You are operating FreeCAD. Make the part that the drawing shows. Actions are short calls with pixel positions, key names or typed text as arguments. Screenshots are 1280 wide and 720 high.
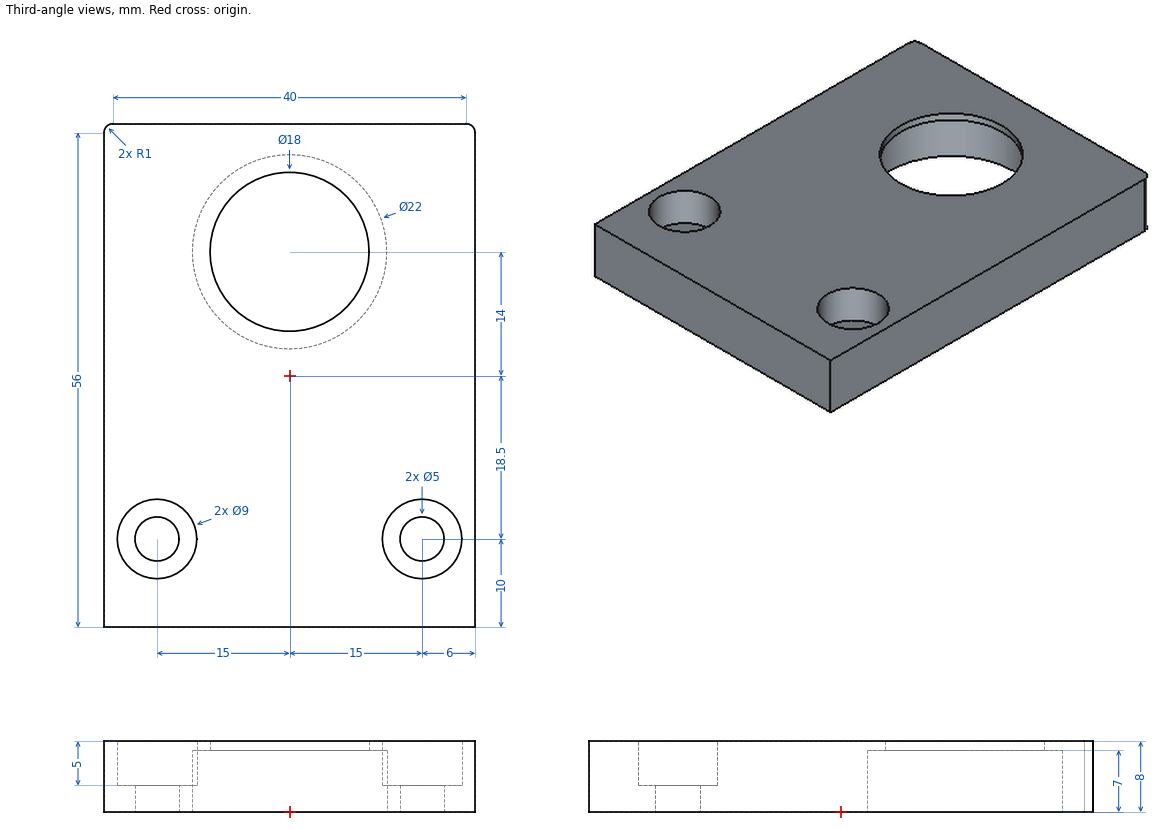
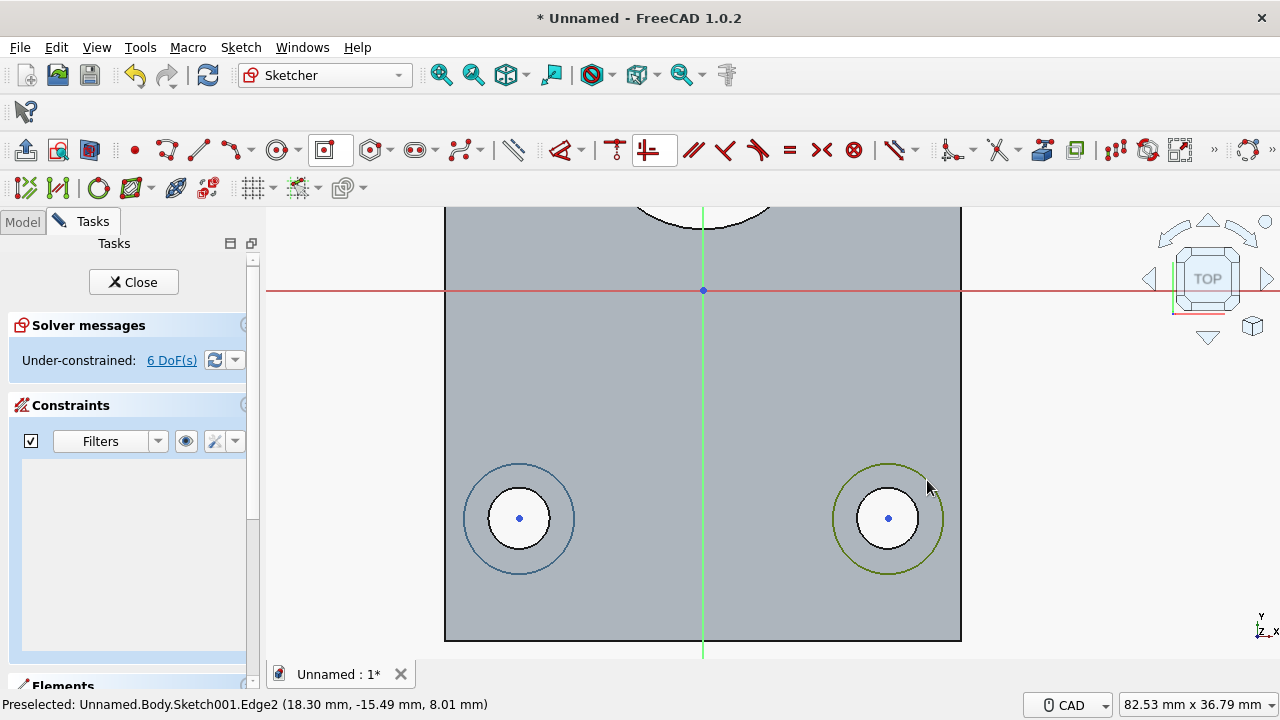
click(790, 150)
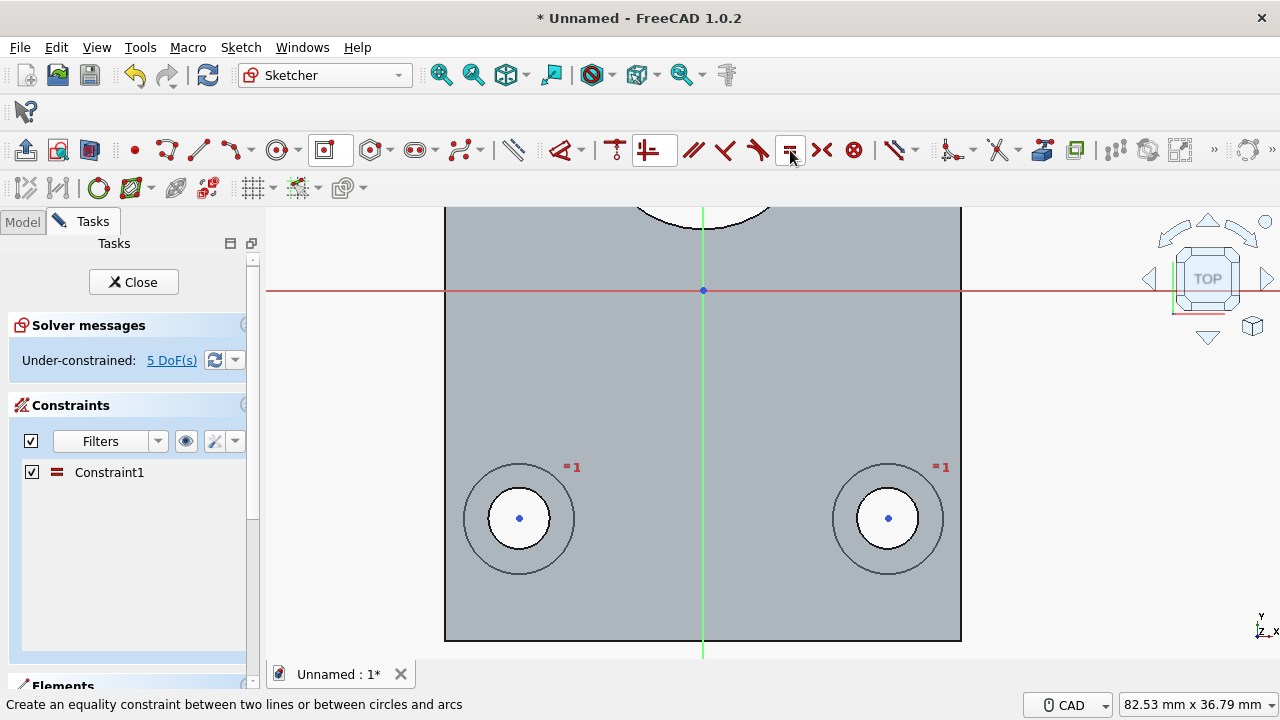
click(519, 519)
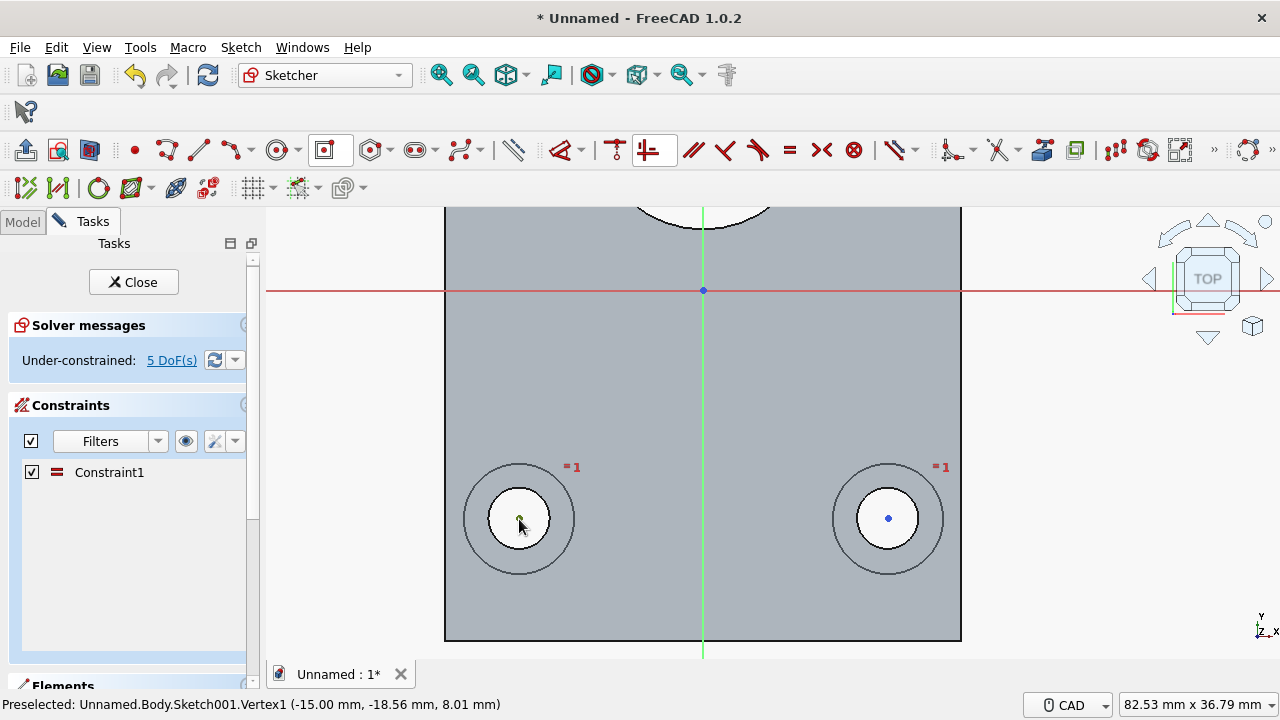
click(888, 519)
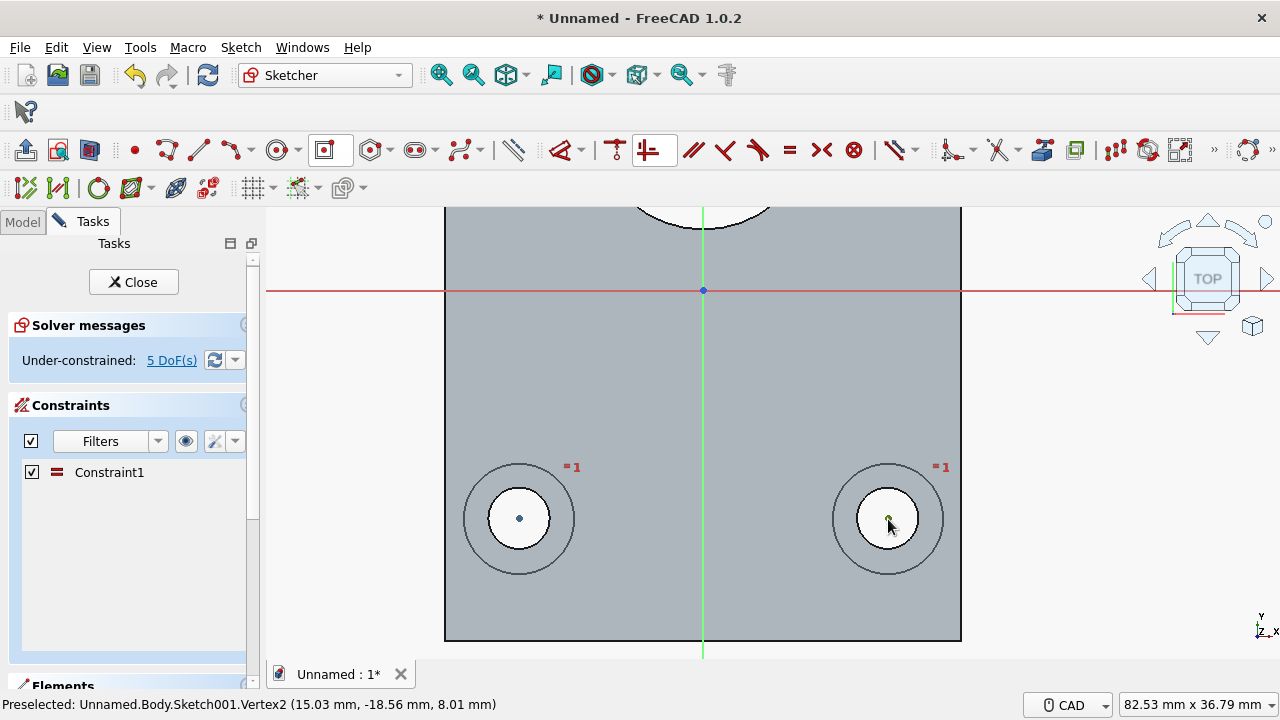
click(672, 150)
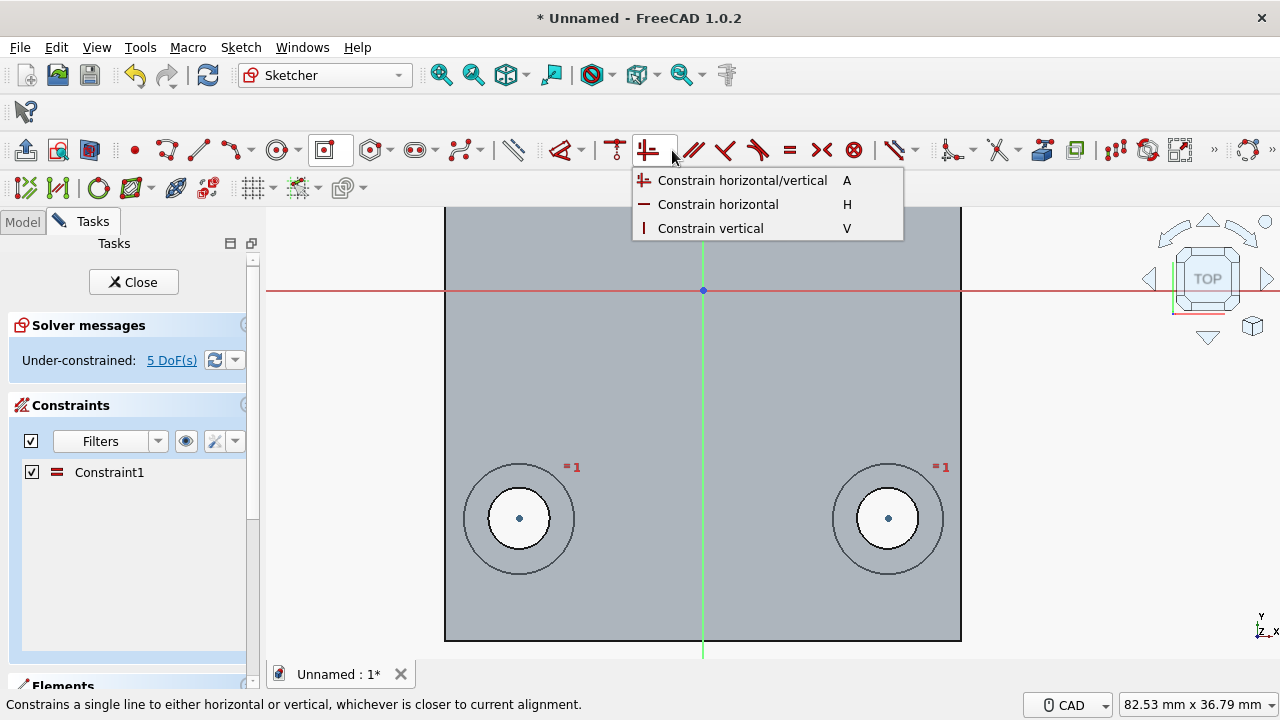
click(768, 204)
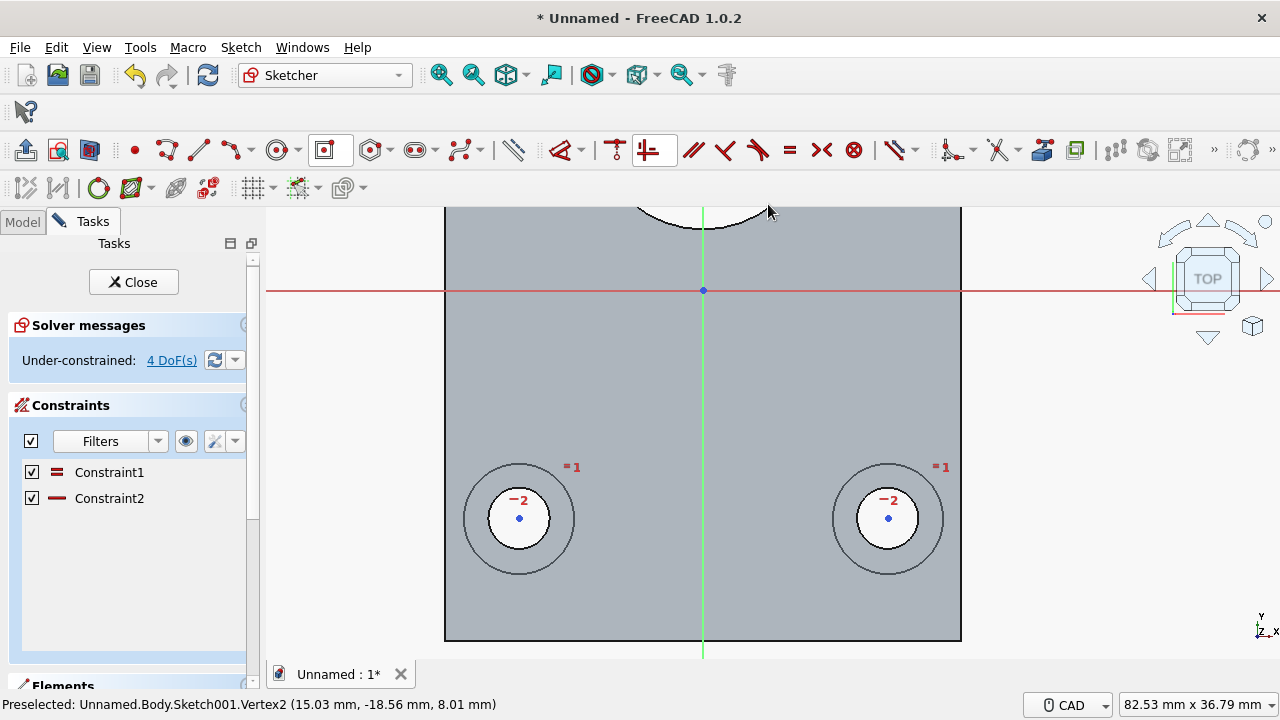
click(560, 150)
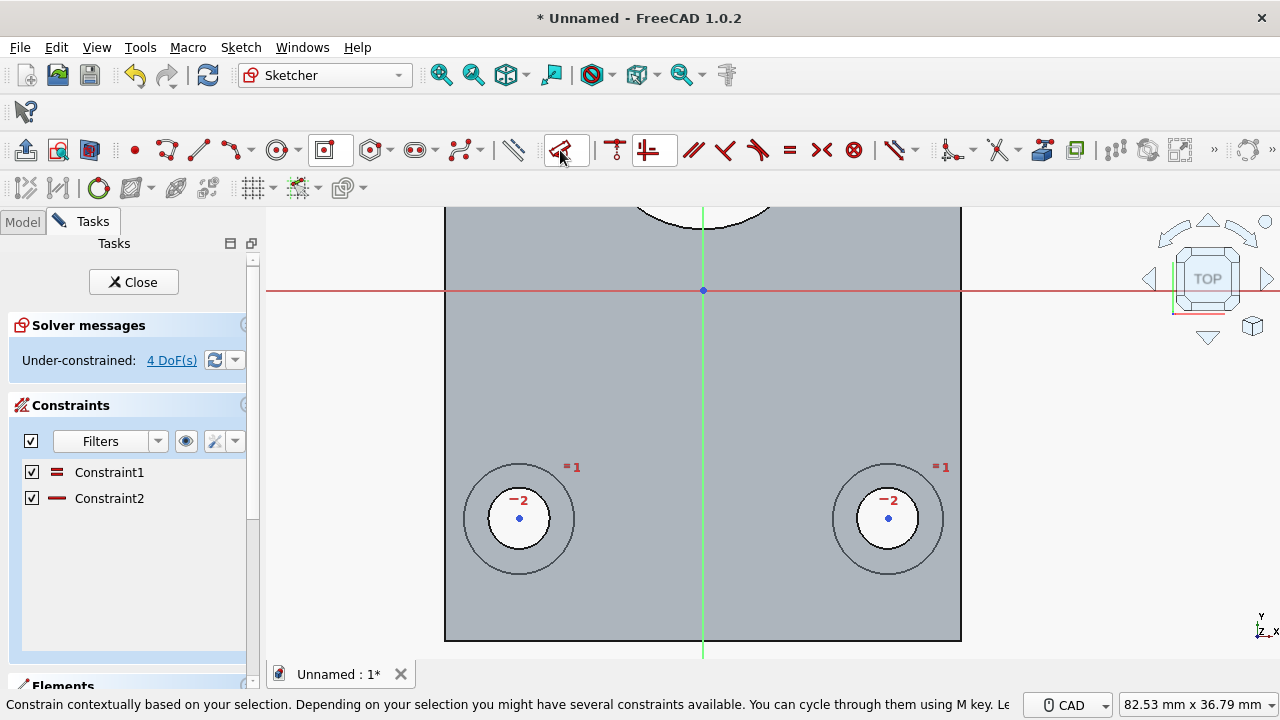
click(558, 480)
click(581, 457)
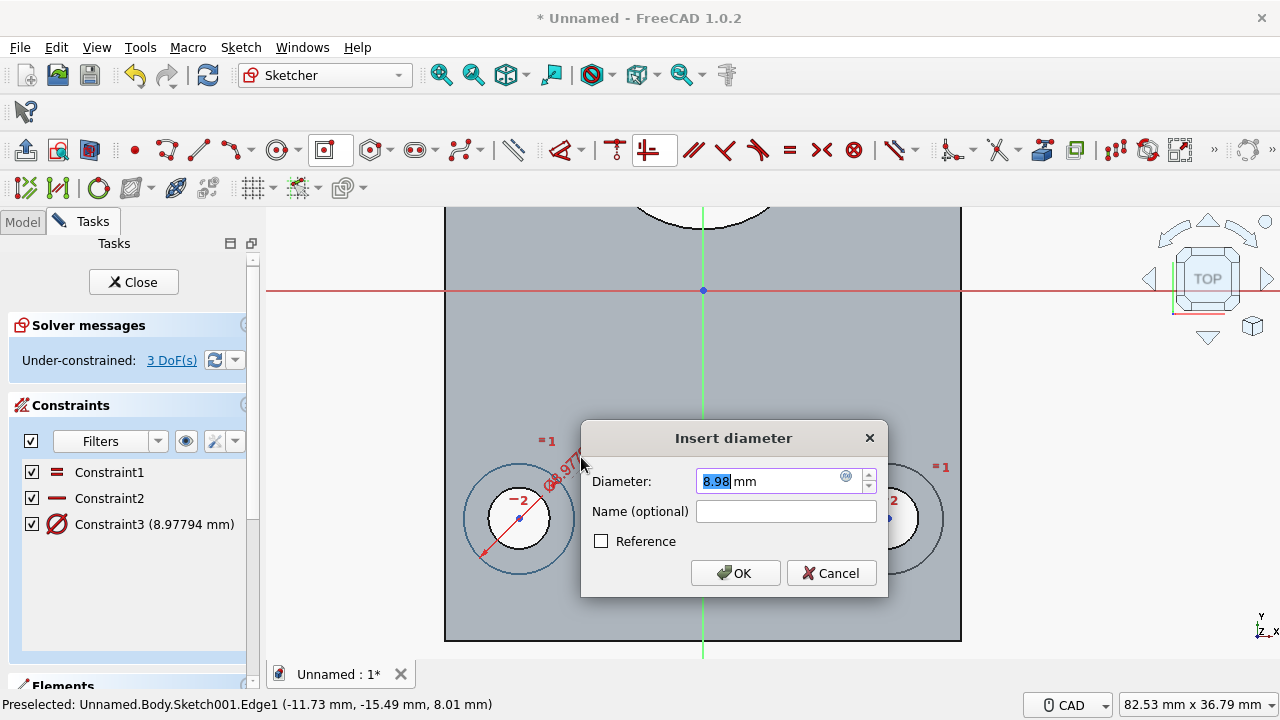
text(9)
key(Return)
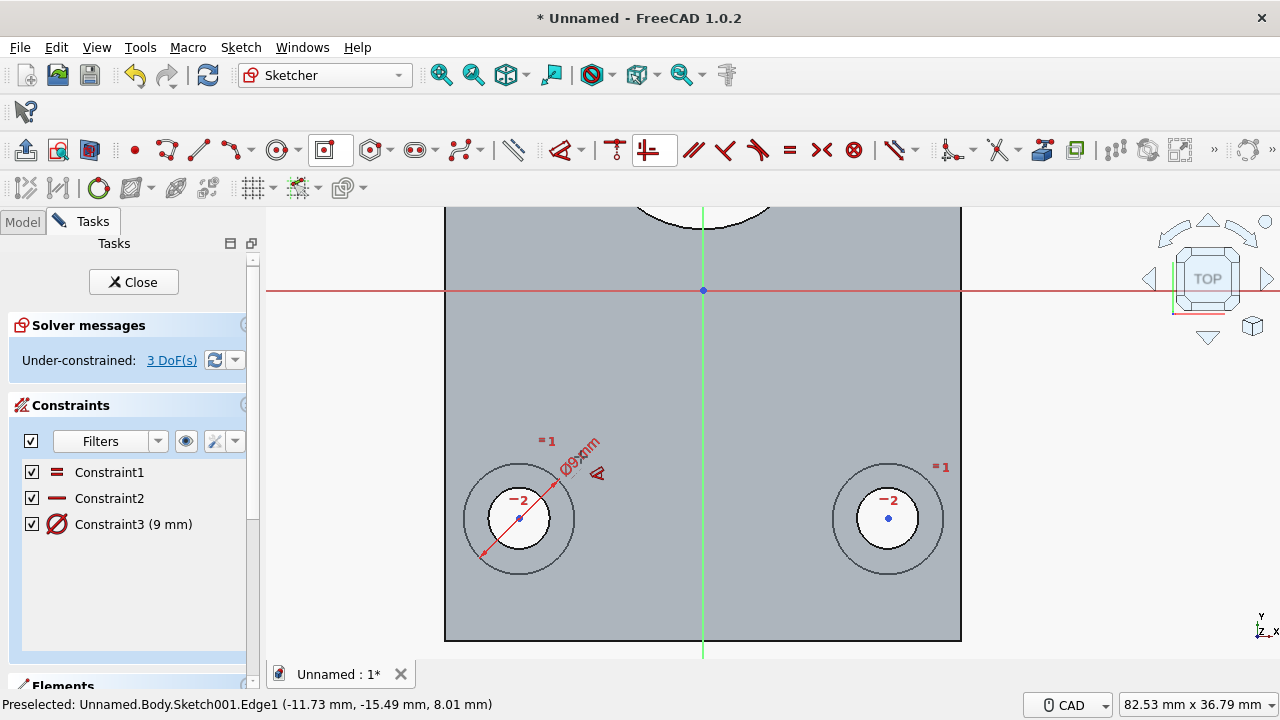
click(519, 519)
click(611, 257)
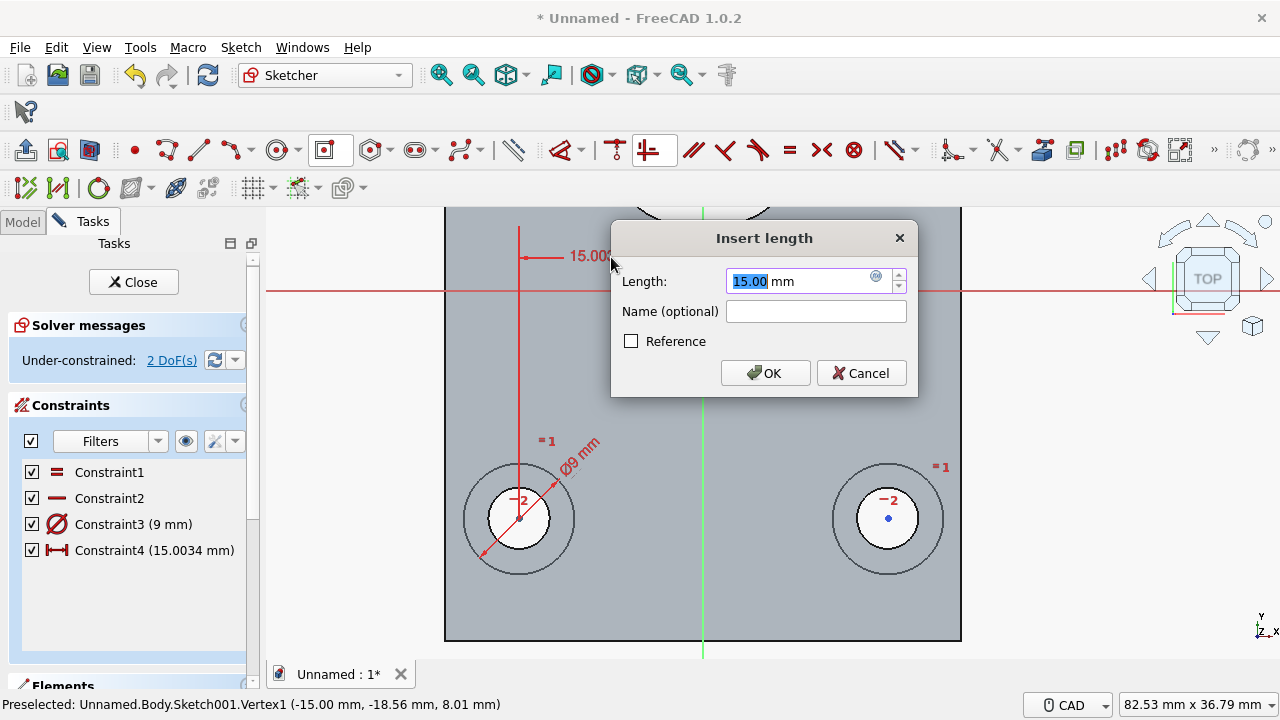
text(15)
key(Return)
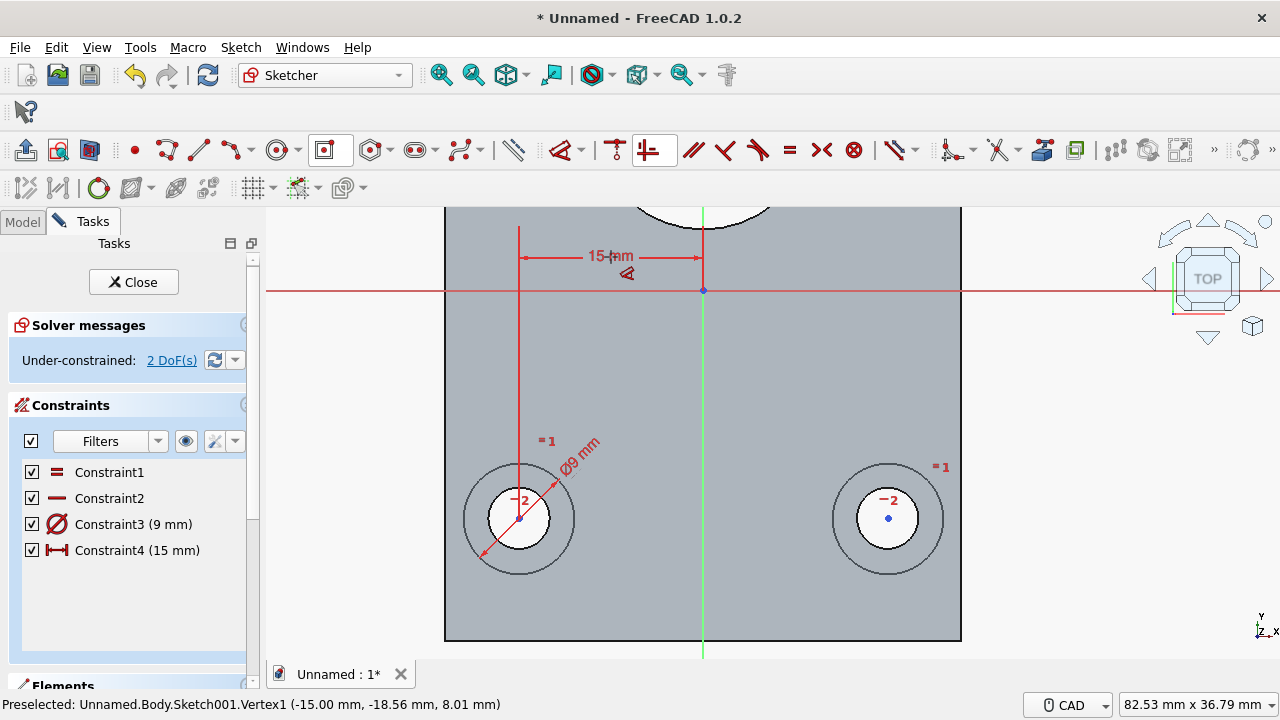
click(888, 519)
click(796, 257)